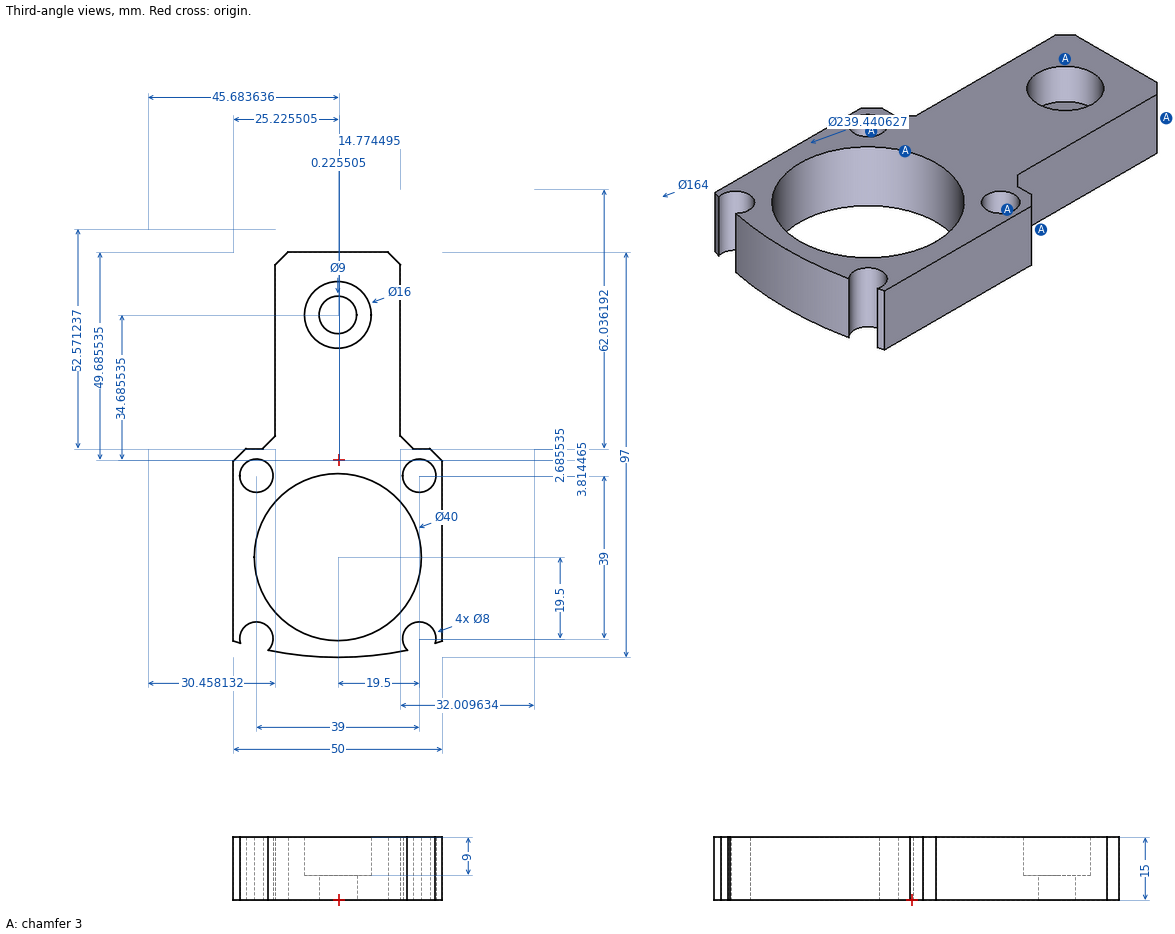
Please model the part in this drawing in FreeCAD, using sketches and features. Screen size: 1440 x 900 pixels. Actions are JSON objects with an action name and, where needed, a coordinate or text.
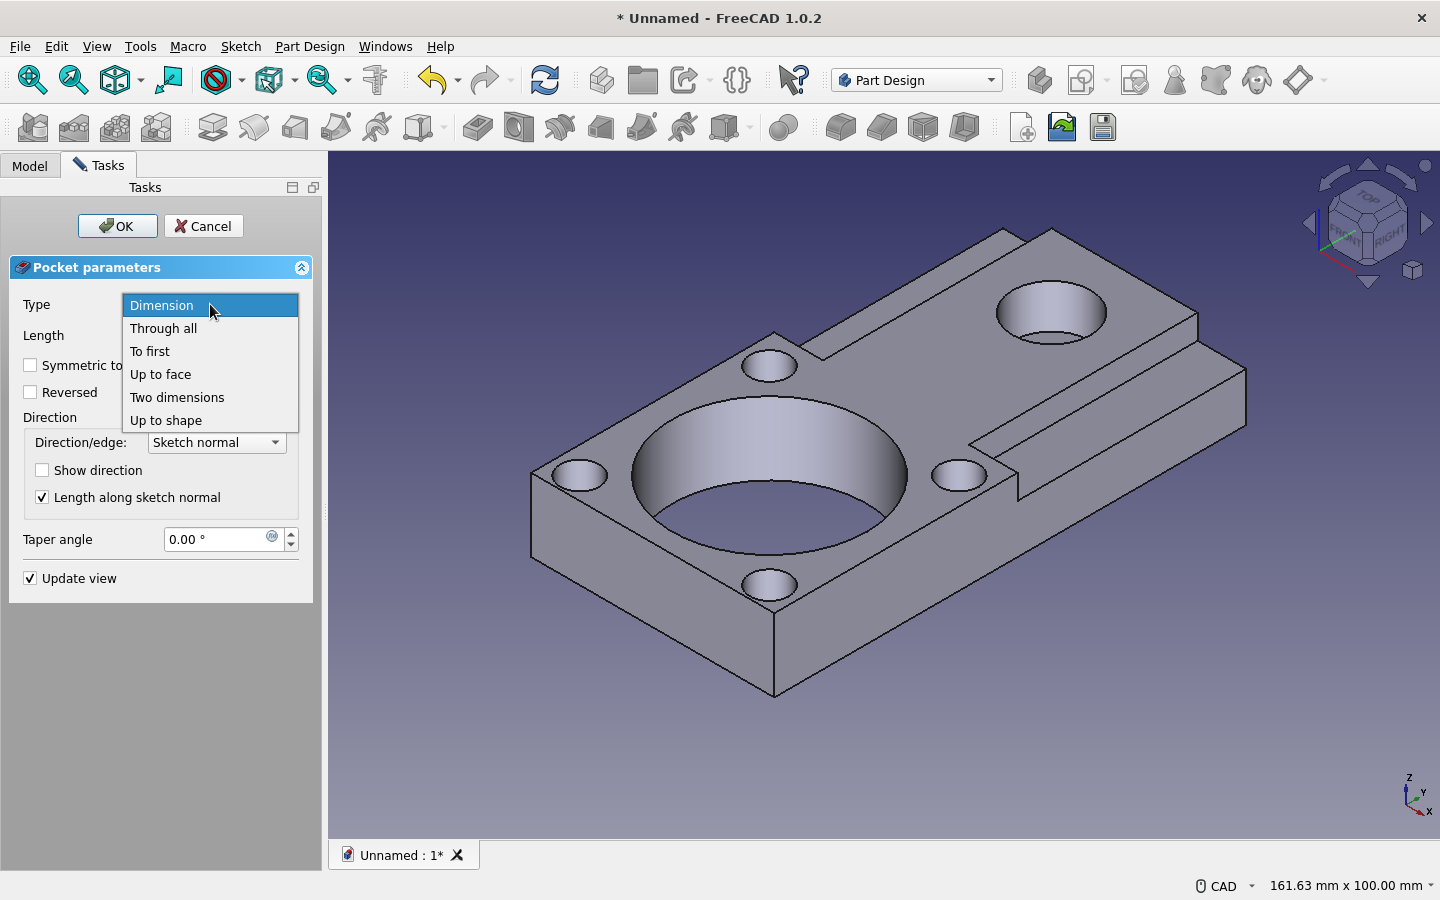
{"action": "left_click", "coordinate": [208, 328]}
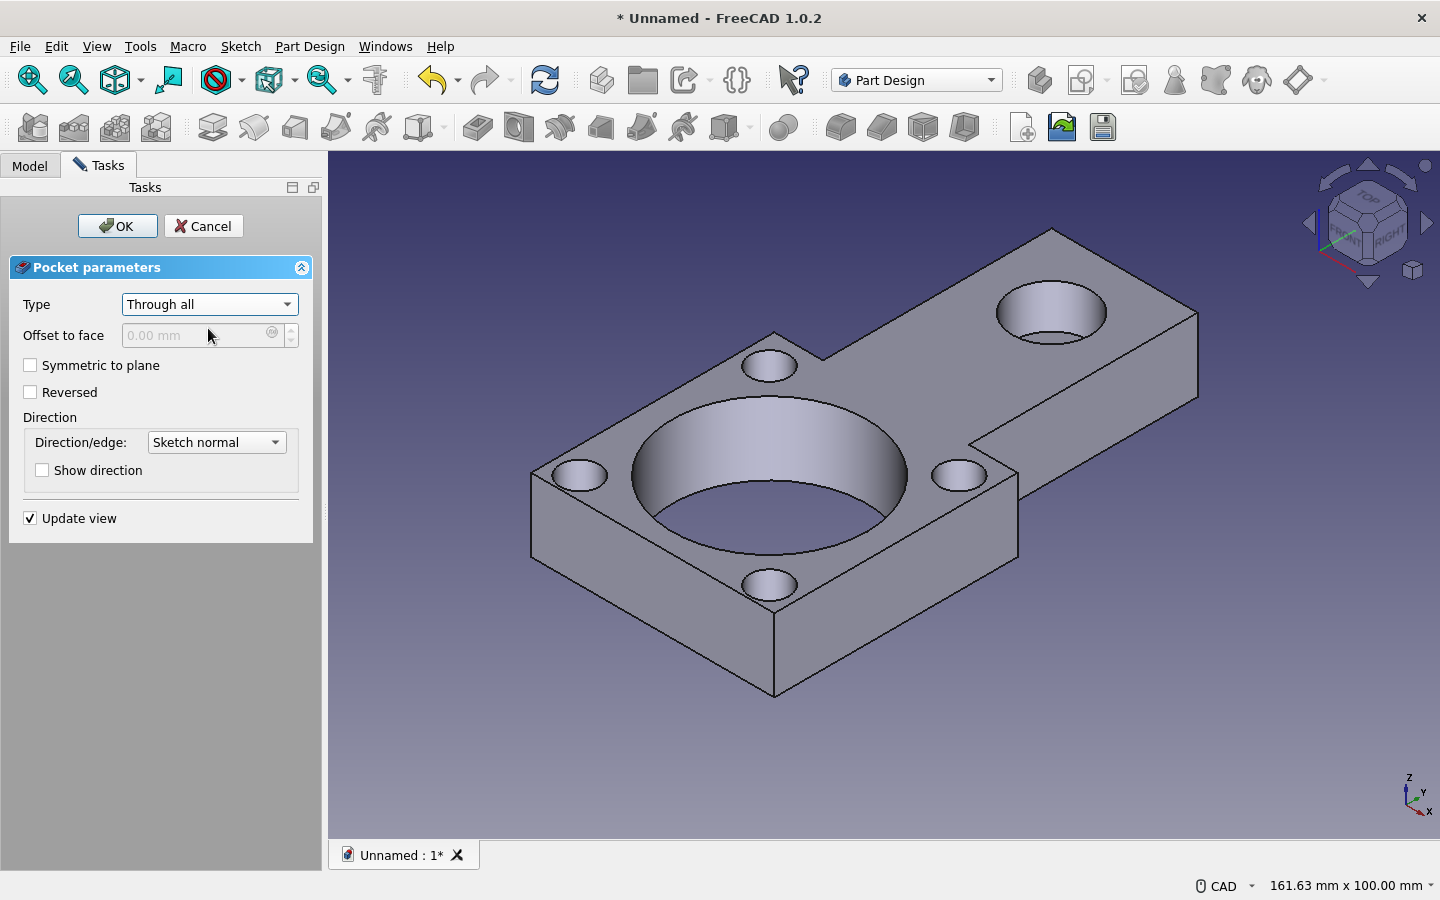
{"action": "left_click", "coordinate": [118, 226]}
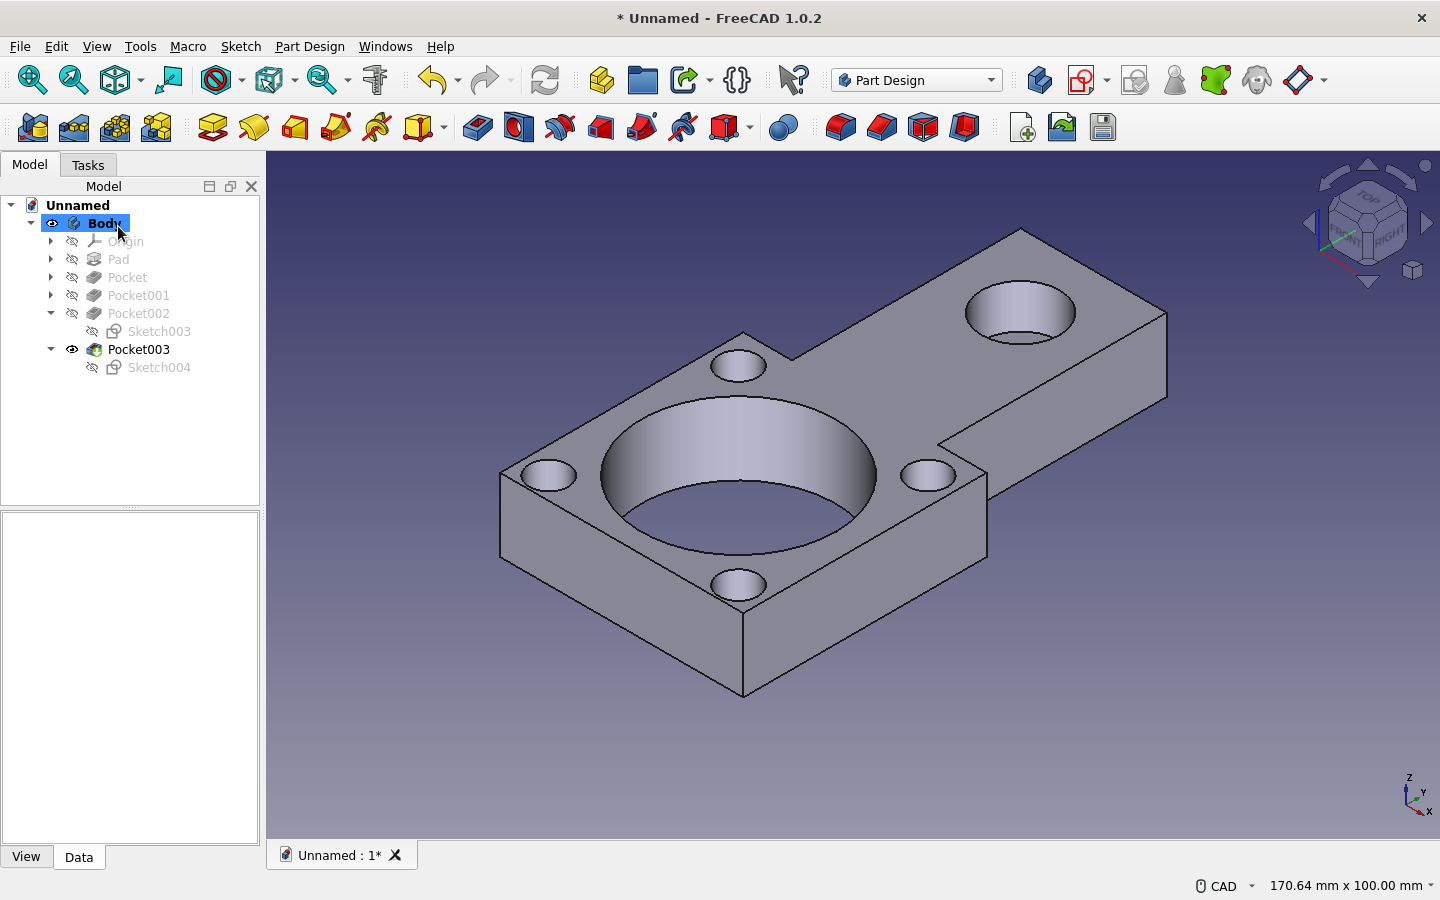
{"action": "key", "text": "2"}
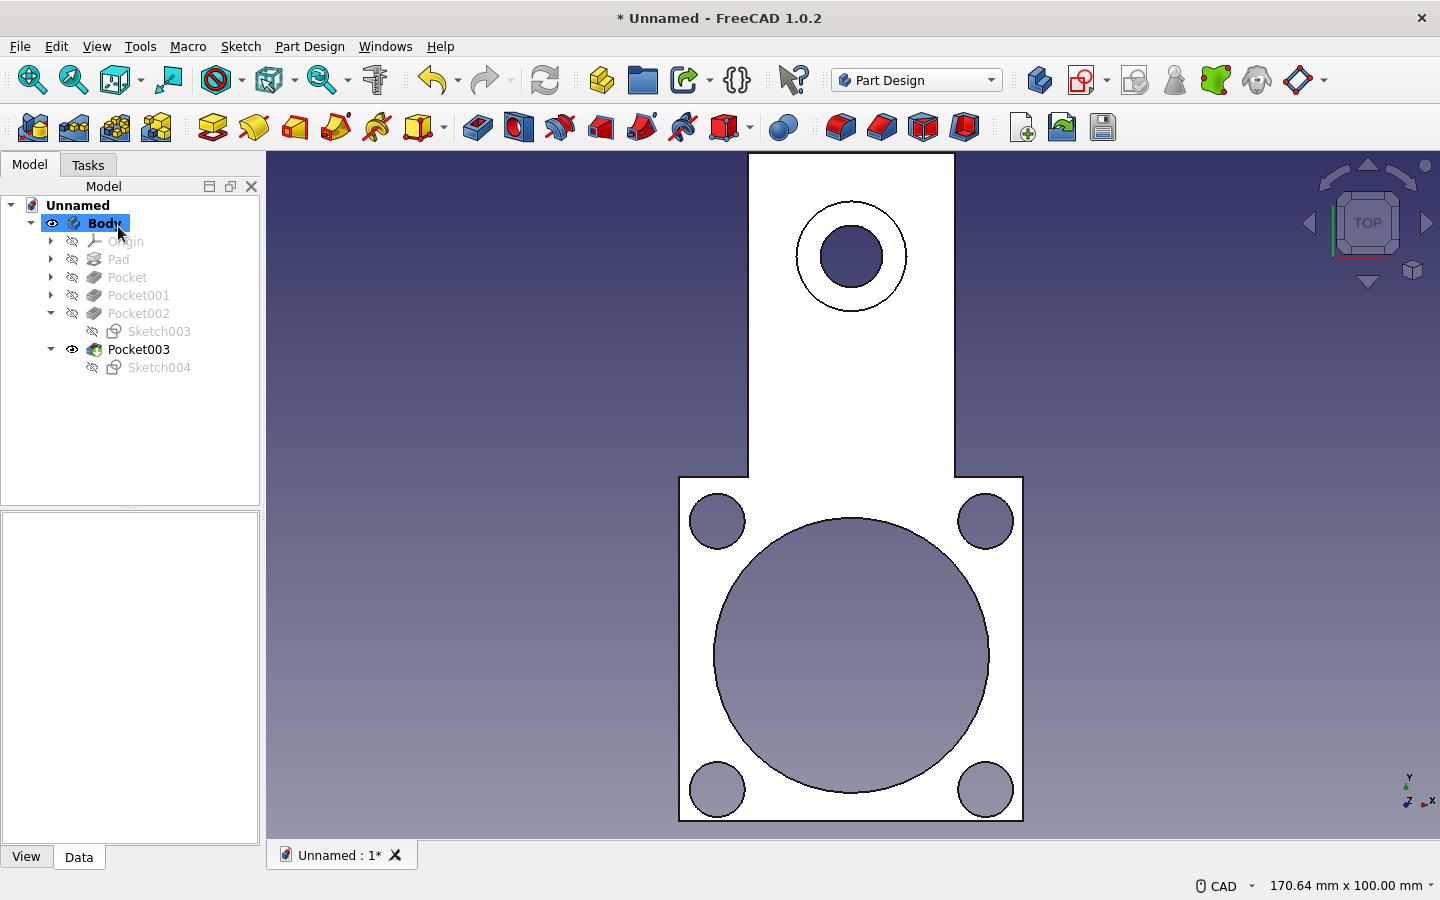
{"action": "key", "text": "0"}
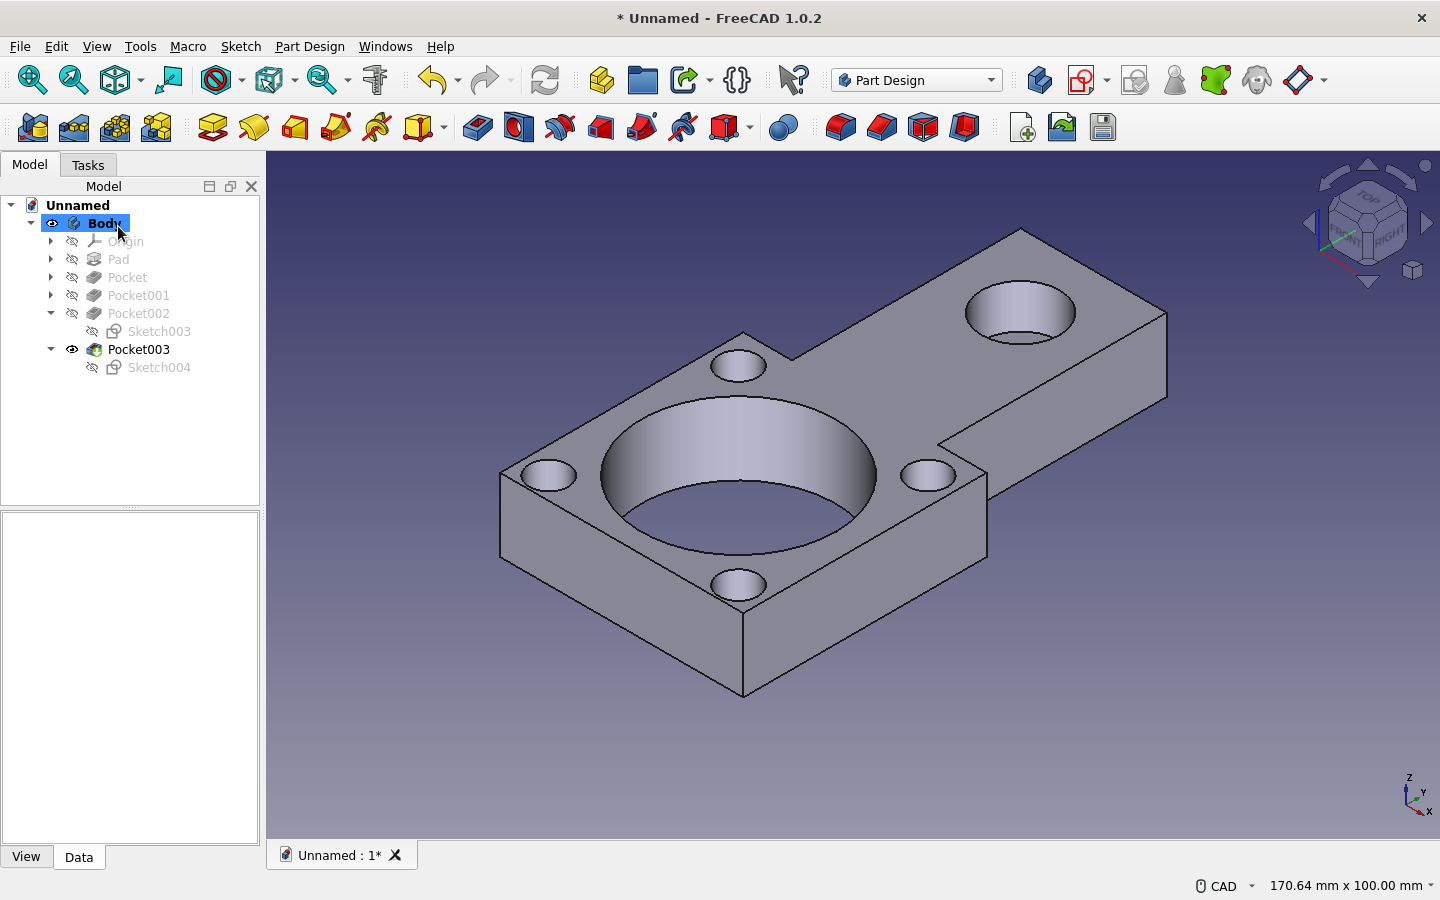
{"action": "key", "text": "1"}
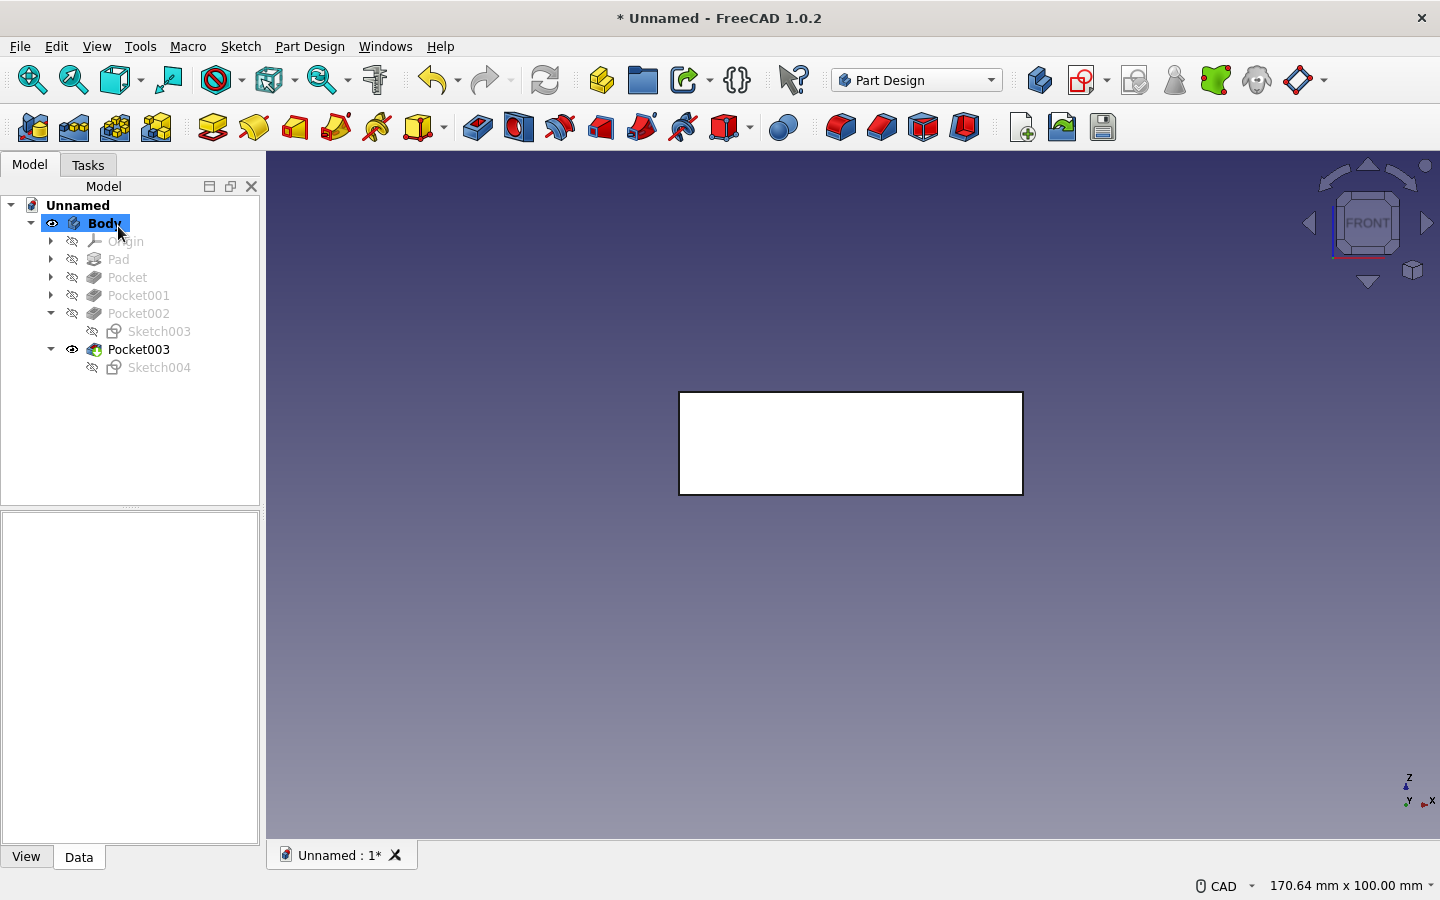
{"action": "left_click", "coordinate": [33, 80]}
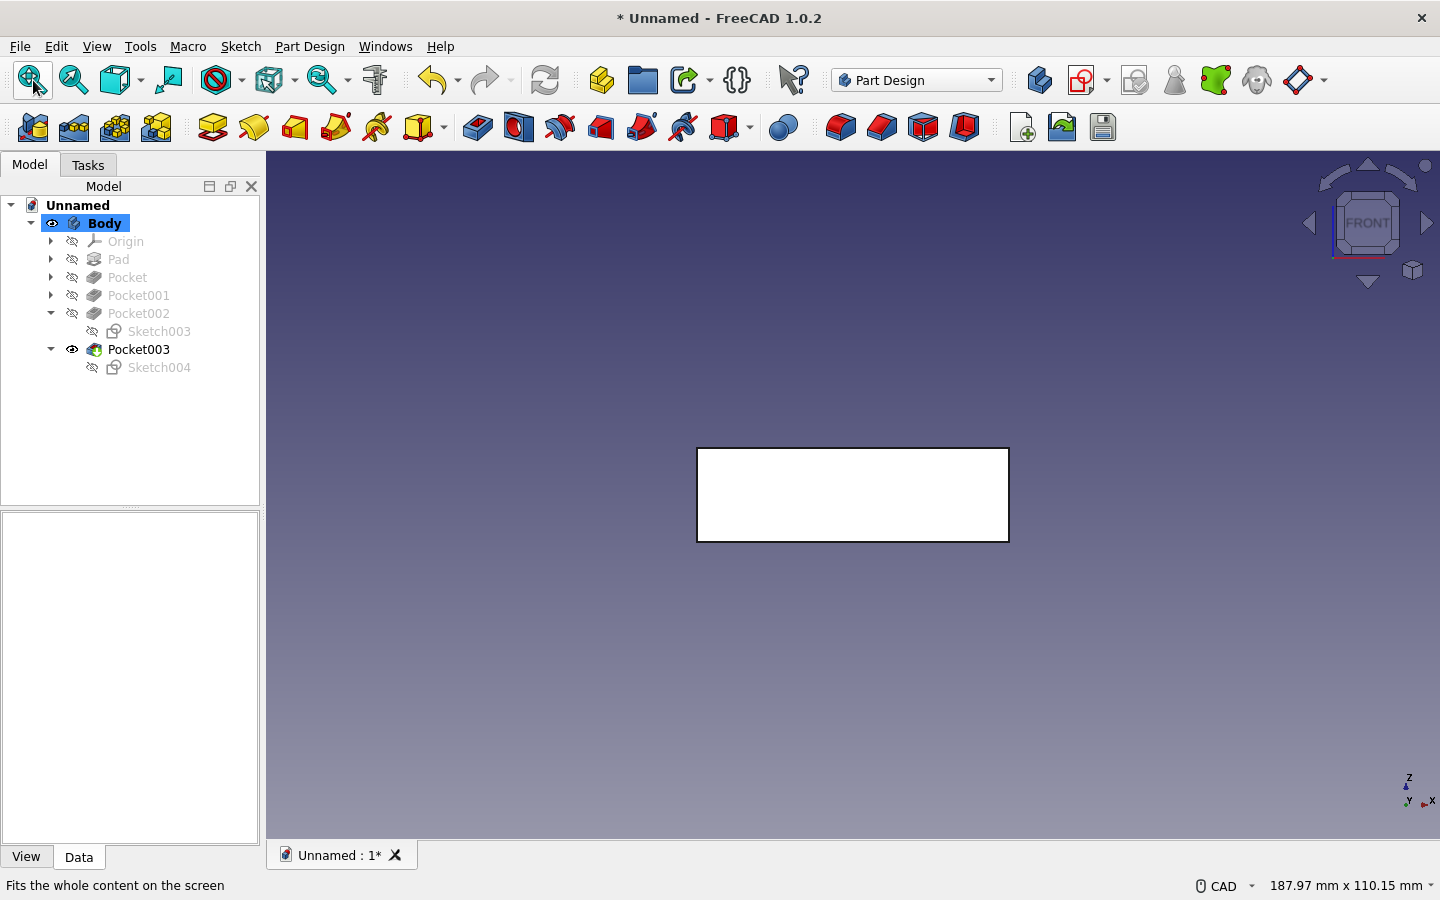
{"action": "key", "text": "3"}